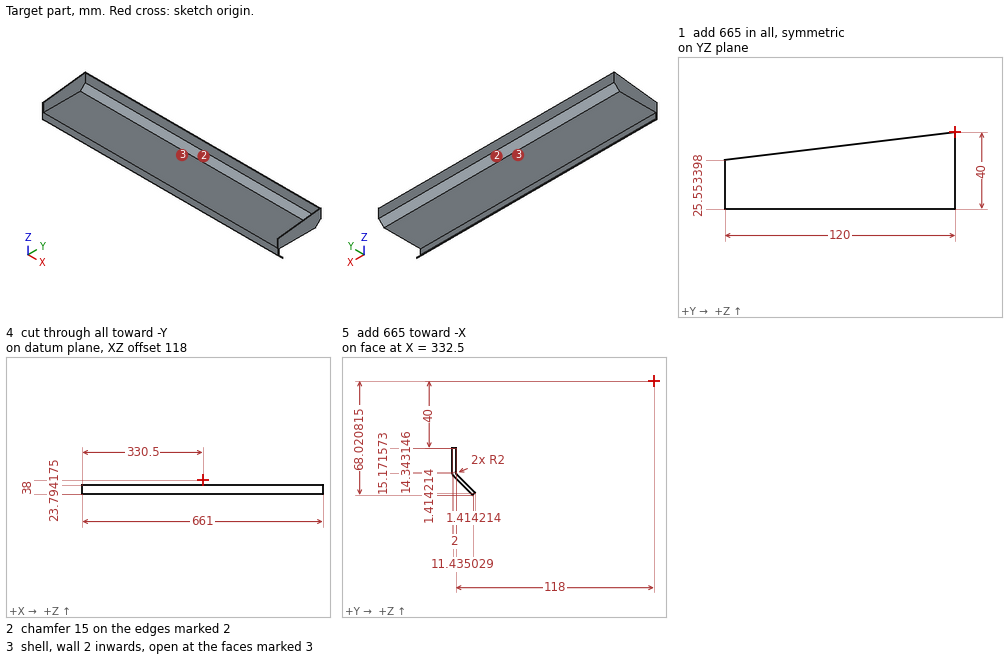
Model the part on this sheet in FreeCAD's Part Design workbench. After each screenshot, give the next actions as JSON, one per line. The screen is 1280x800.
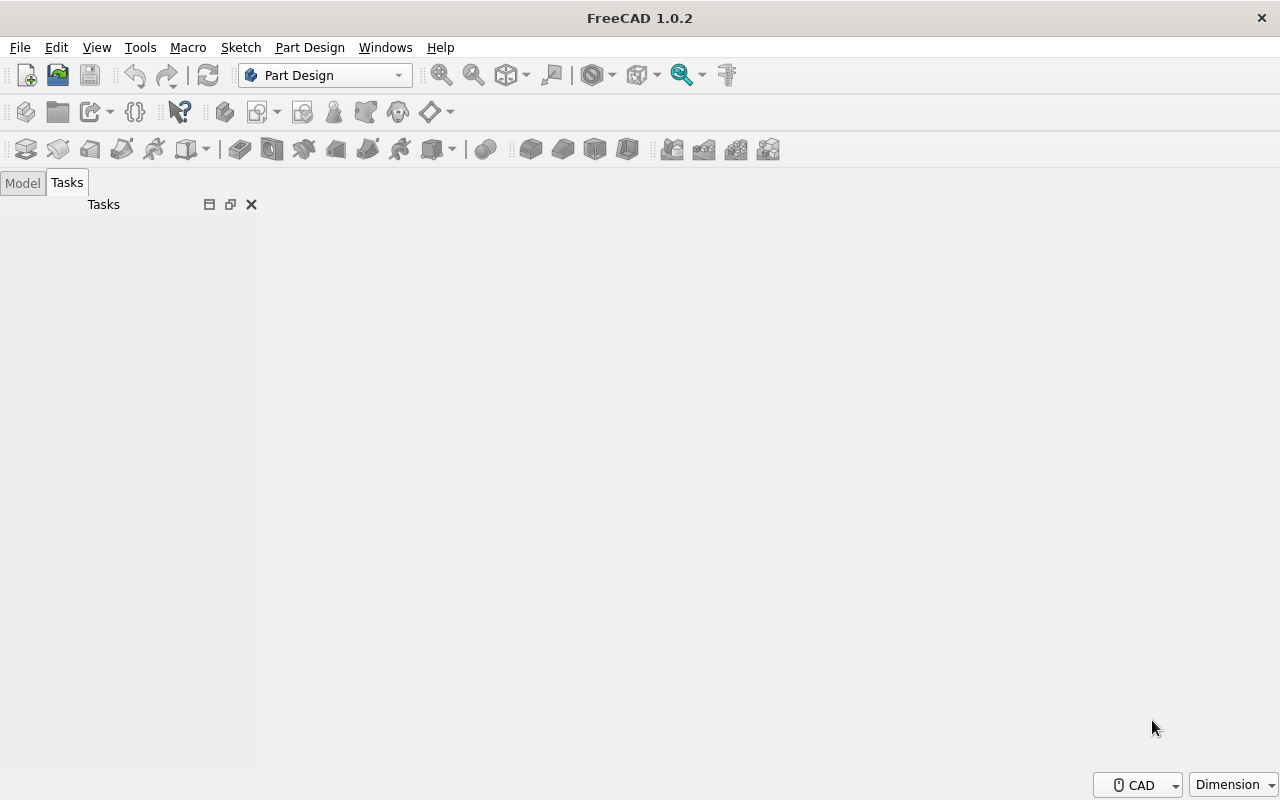
{"action": "key", "text": "ctrl+n"}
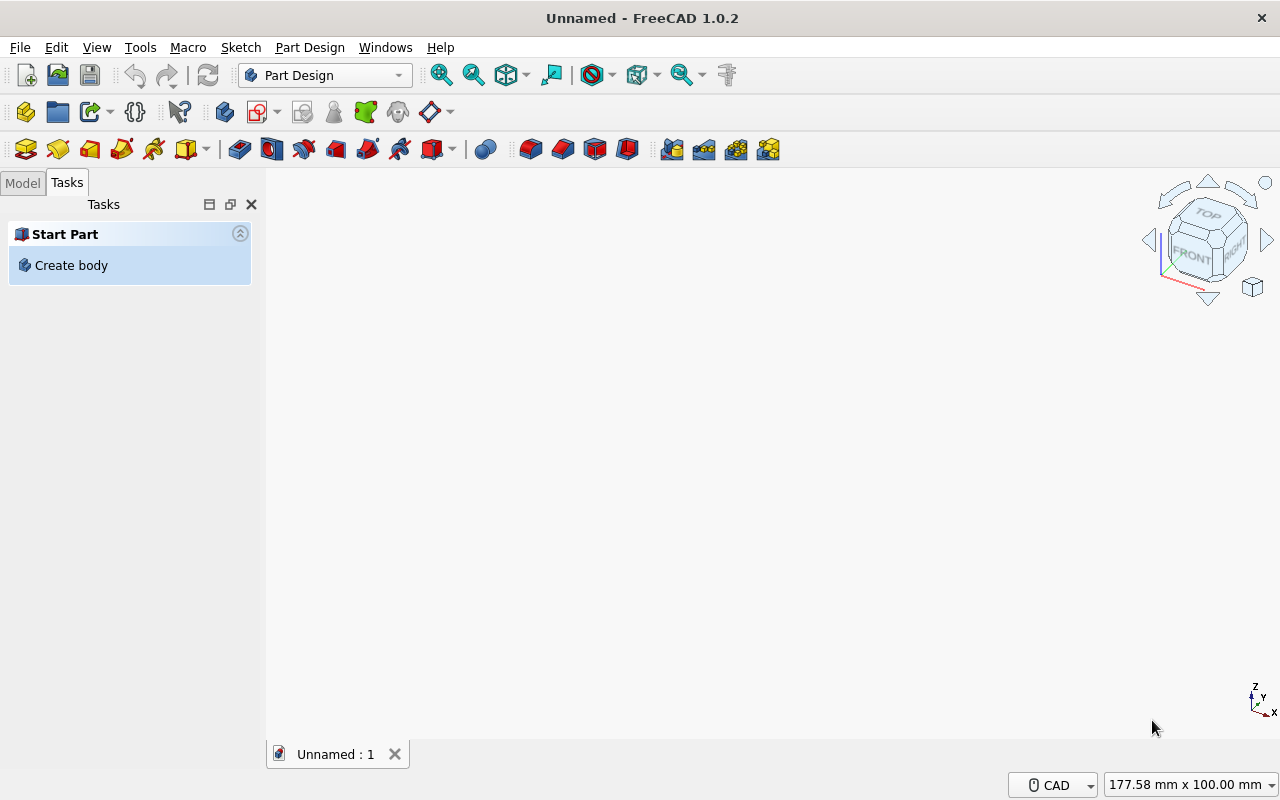
{"action": "left_click", "coordinate": [258, 112]}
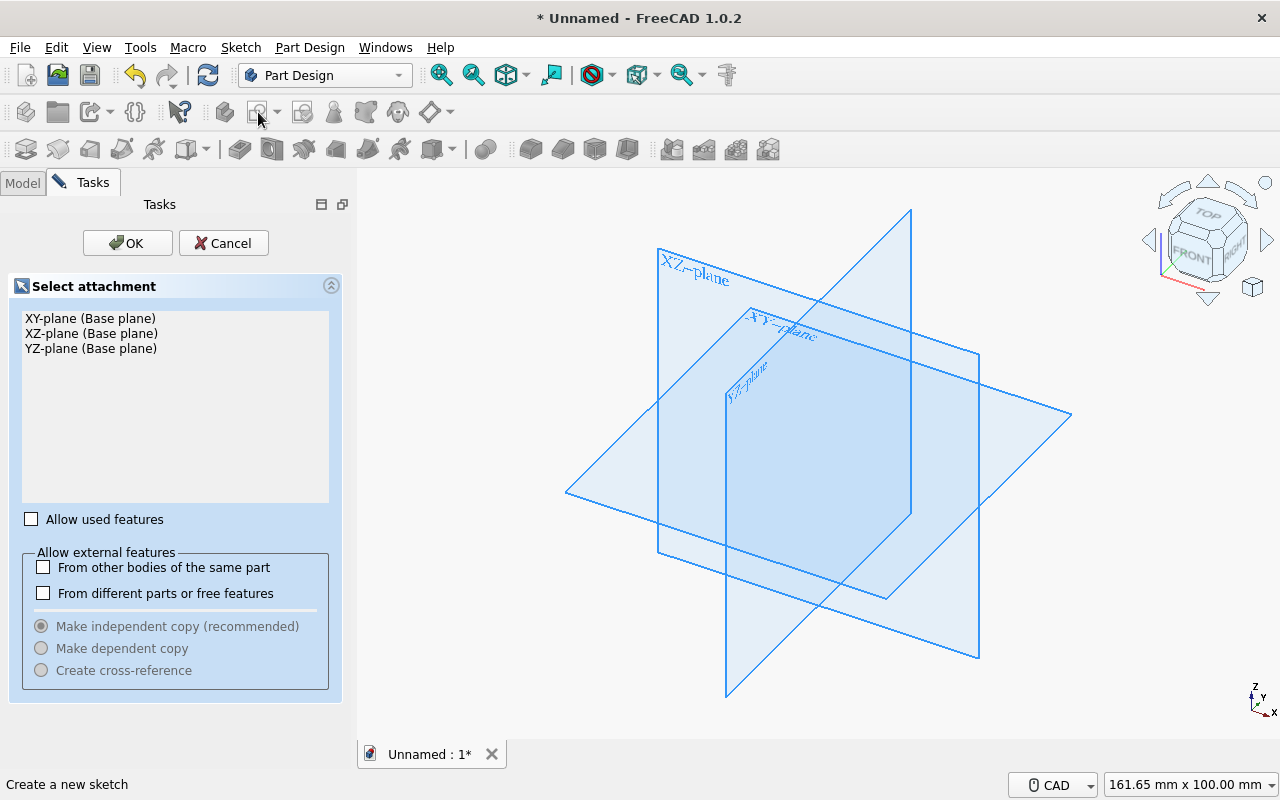
{"action": "left_click", "coordinate": [82, 348]}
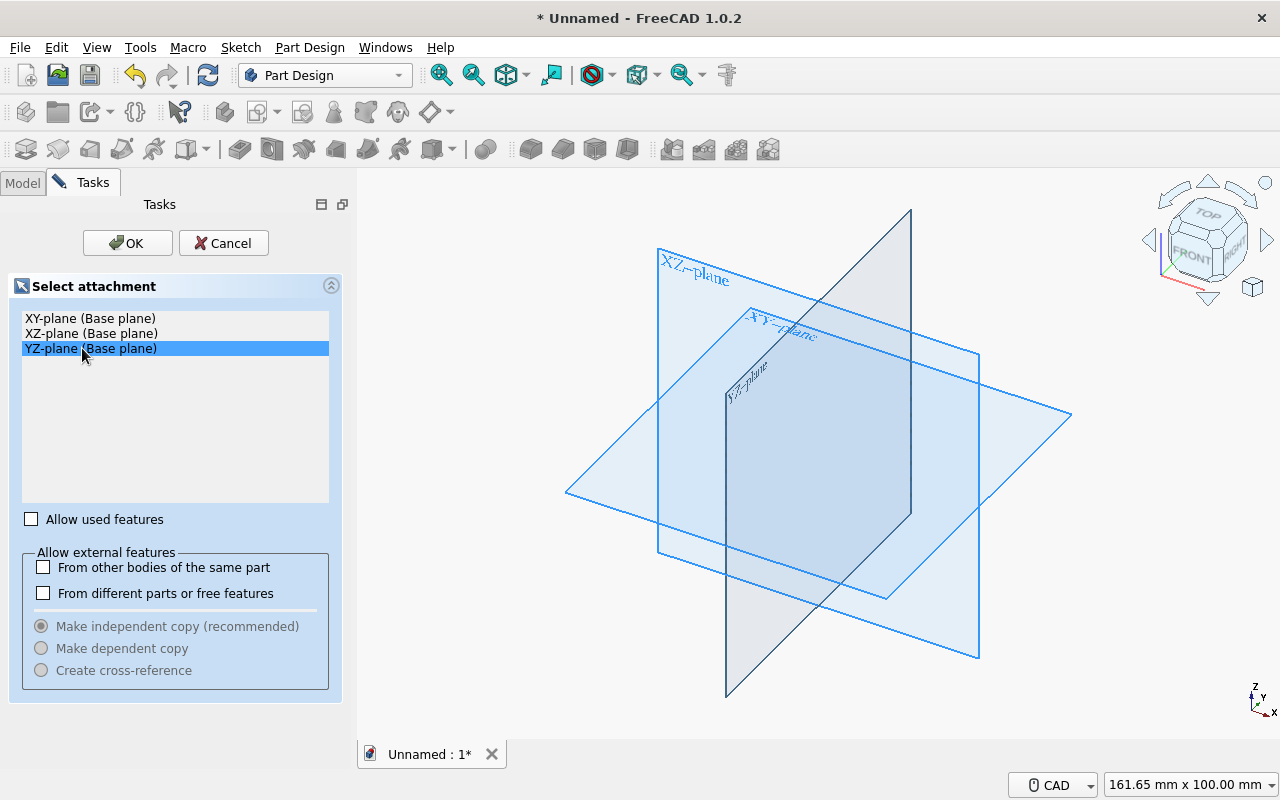
{"action": "left_click", "coordinate": [128, 243]}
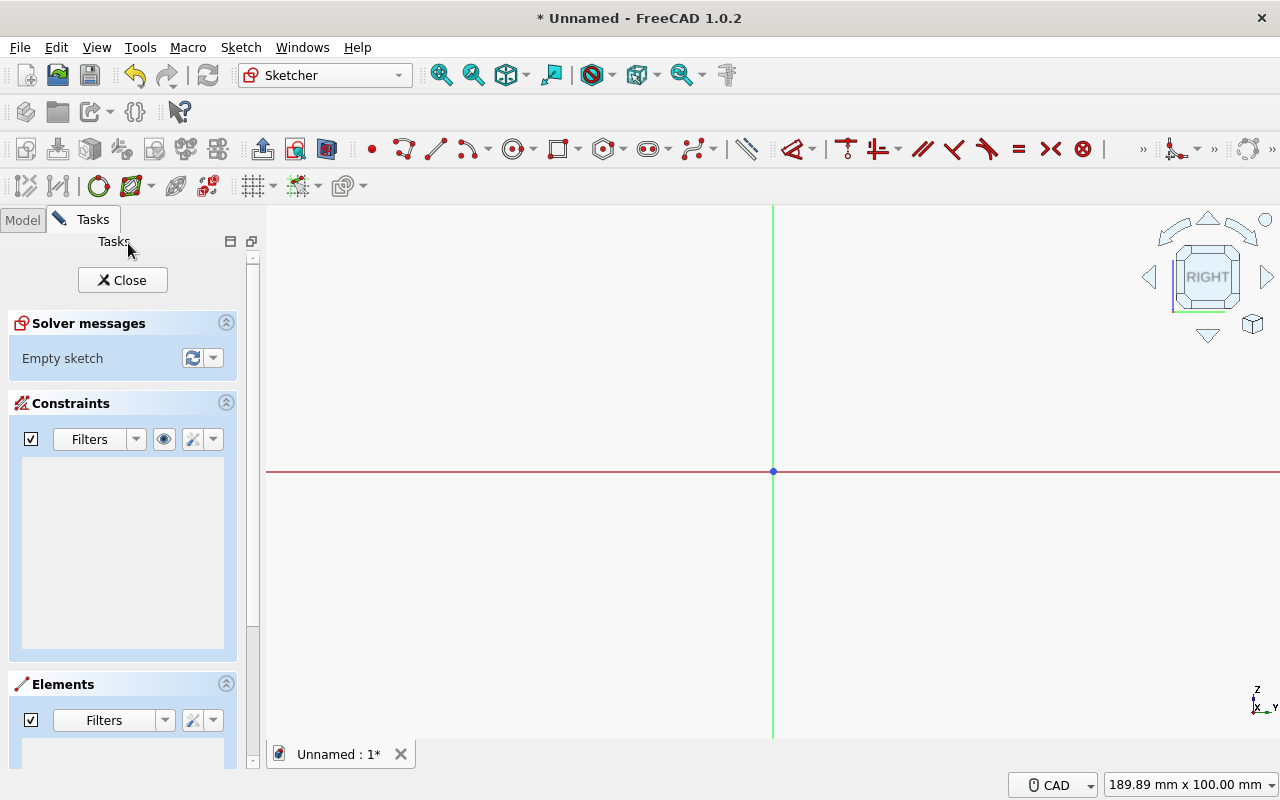
{"action": "scroll", "coordinate": [1115, 255], "scroll_direction": "down", "scroll_amount": 2}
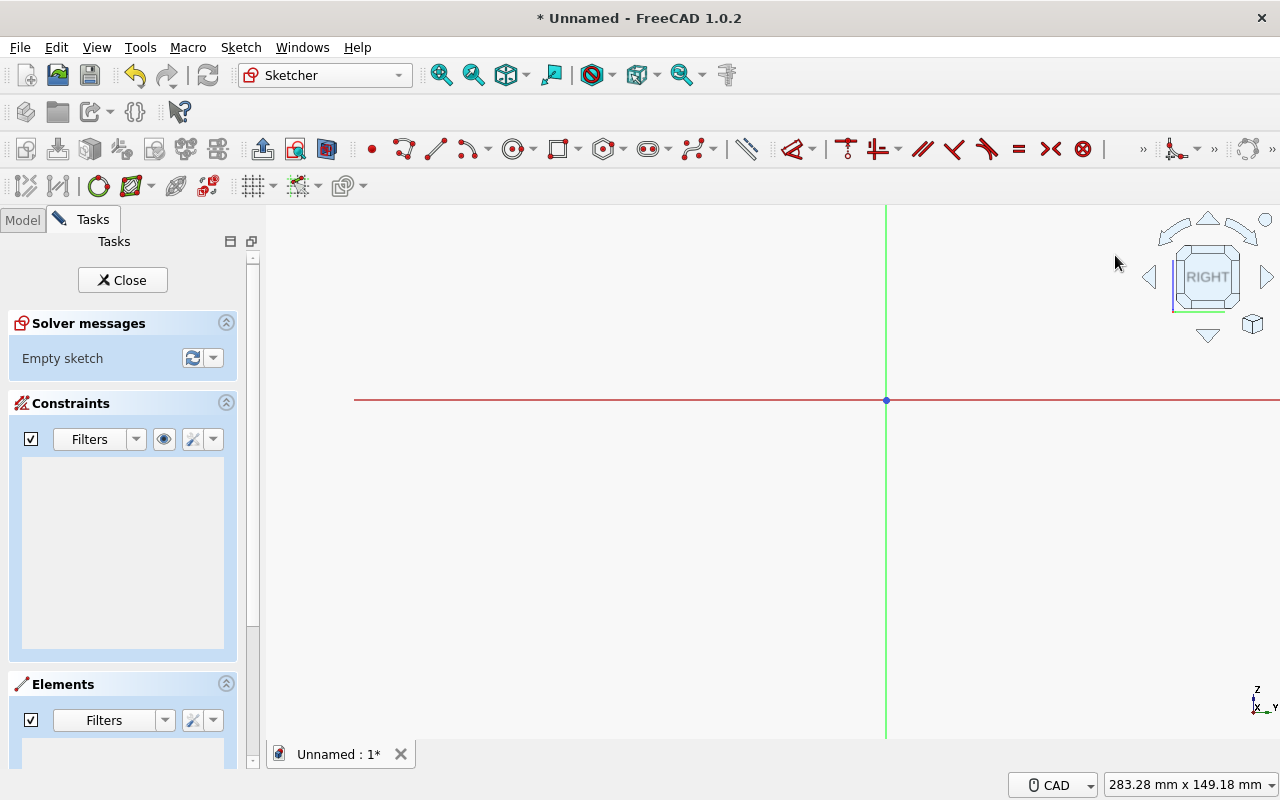
{"action": "key", "text": "g m"}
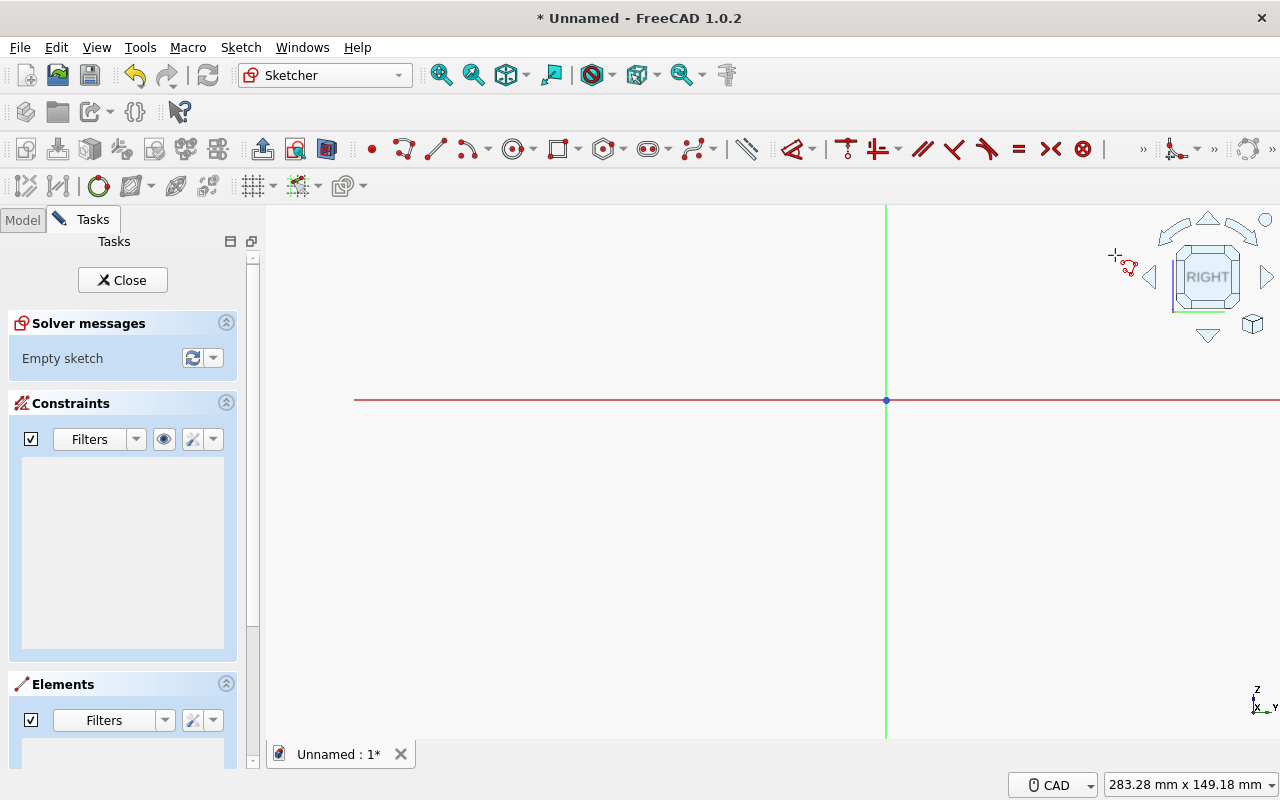
{"action": "left_click", "coordinate": [886, 400]}
{"action": "left_click", "coordinate": [456, 452]}
{"action": "left_click", "coordinate": [456, 544]}
{"action": "left_click", "coordinate": [877, 544]}
{"action": "left_click", "coordinate": [886, 400]}
{"action": "key", "text": "Escape"}
{"action": "key", "text": "Escape"}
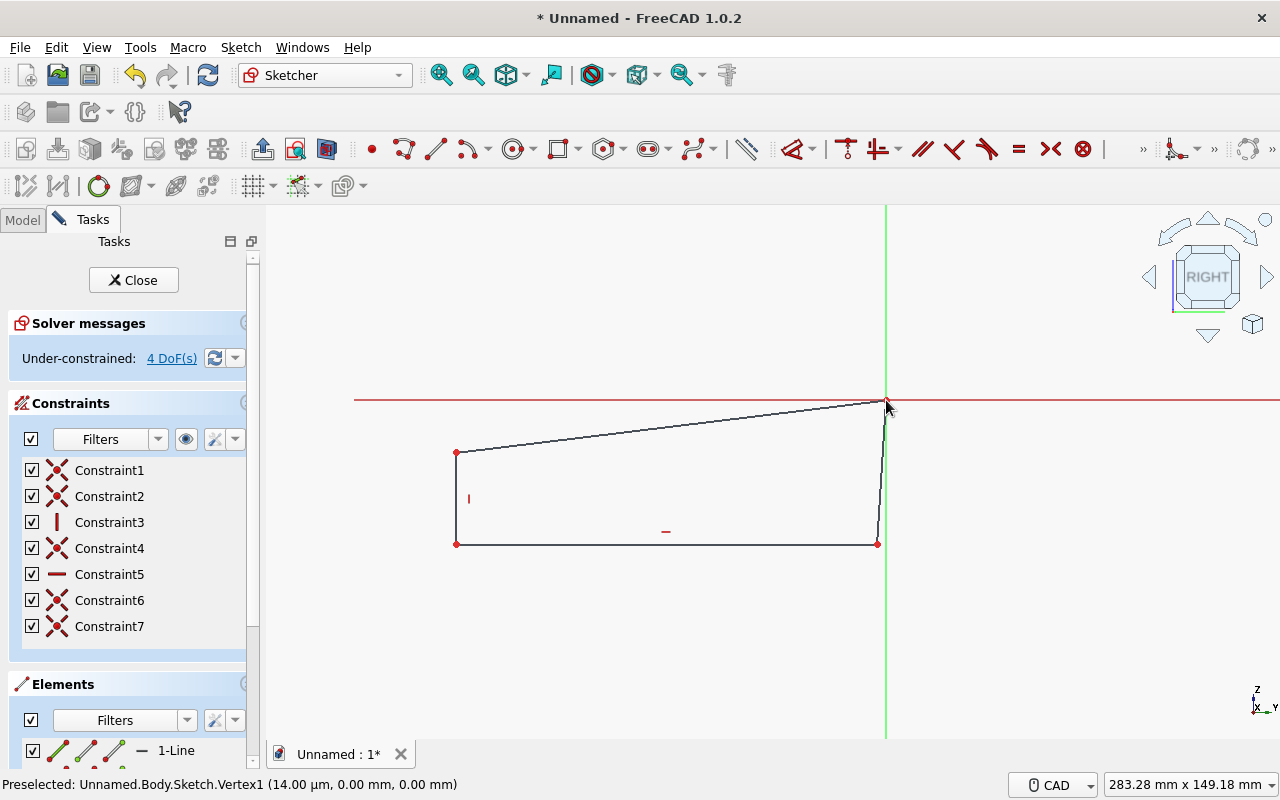
{"action": "left_click", "coordinate": [883, 444]}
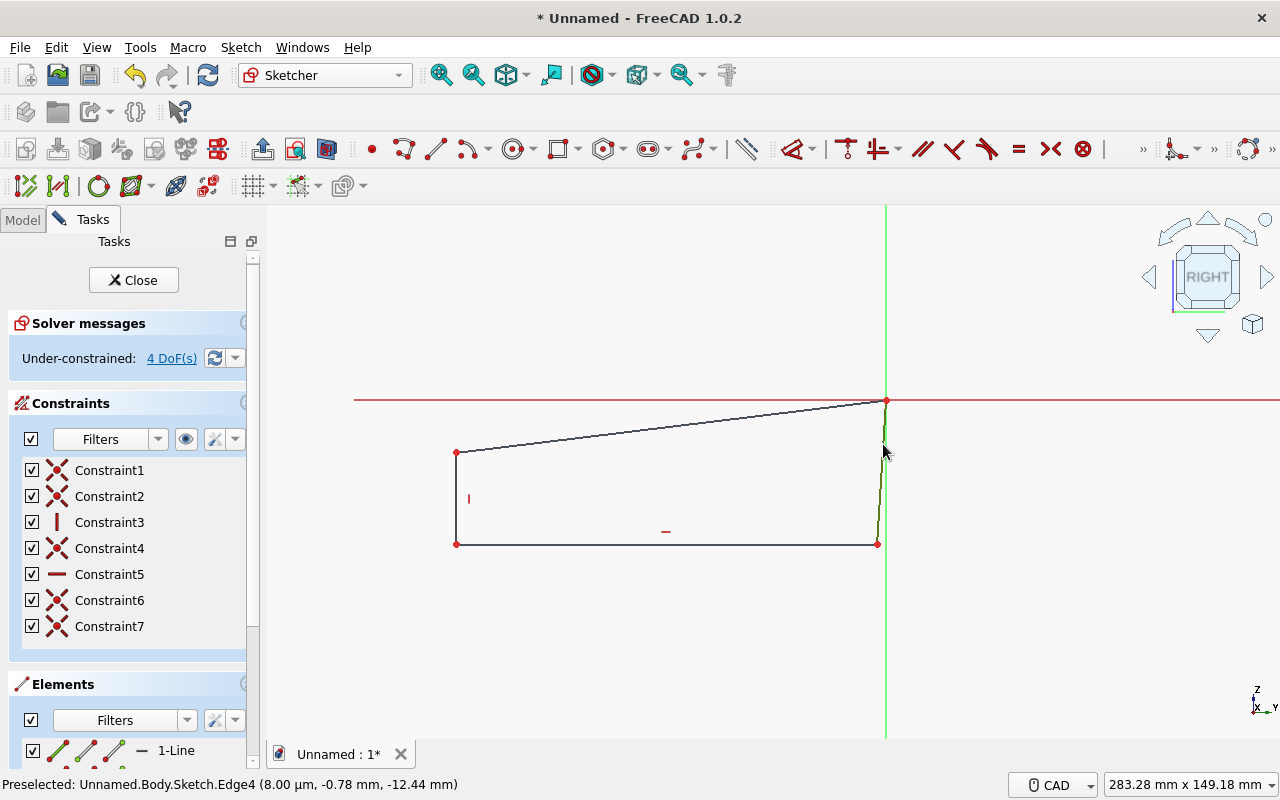
{"action": "key", "text": "v"}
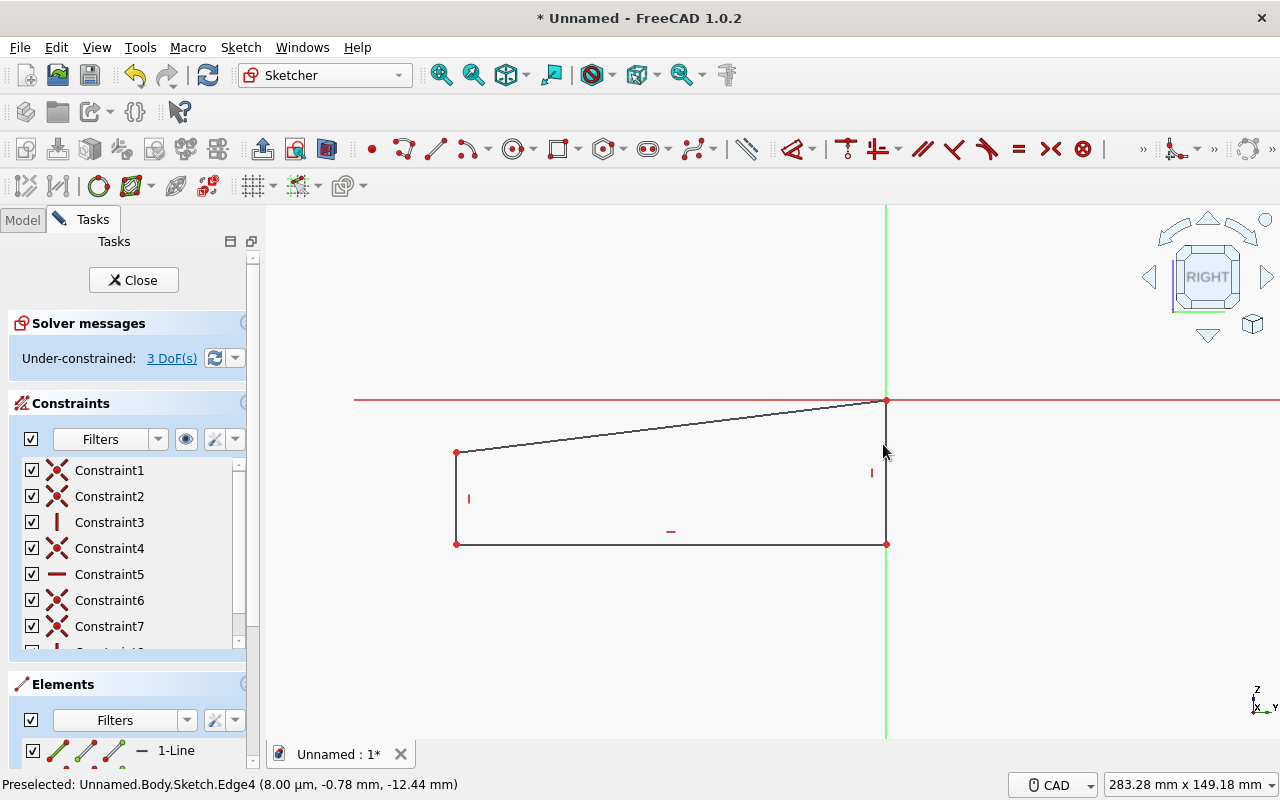
{"action": "key", "text": "d"}